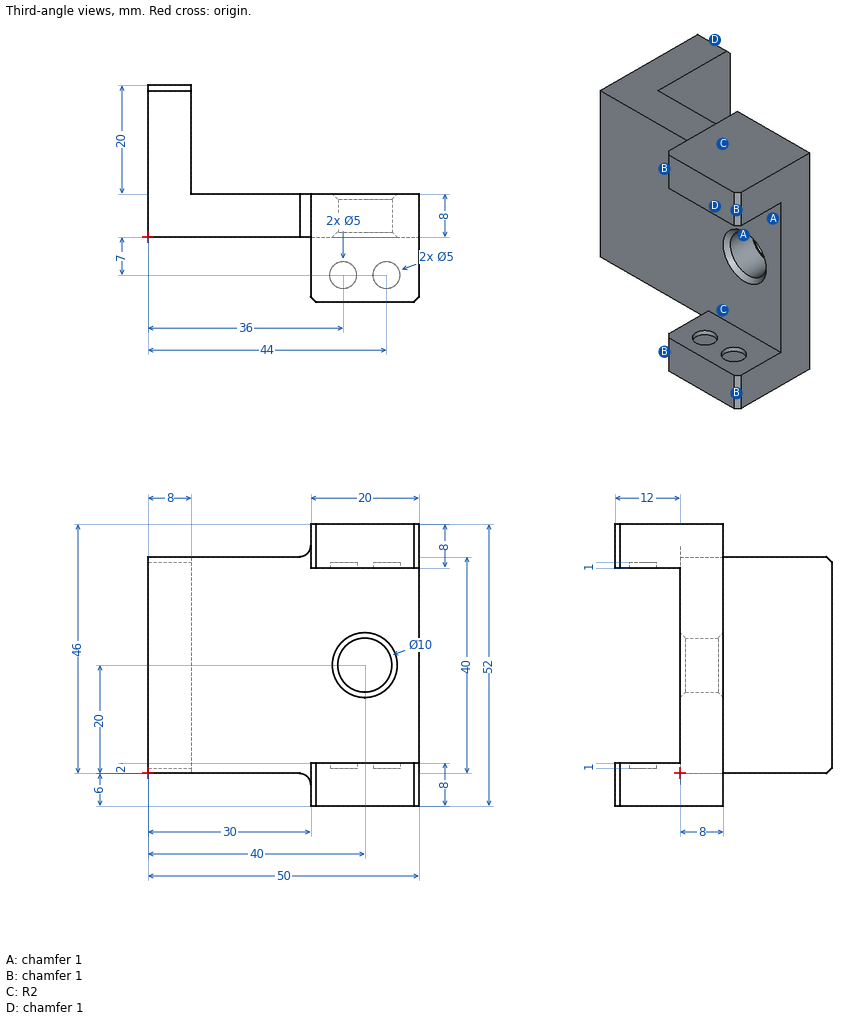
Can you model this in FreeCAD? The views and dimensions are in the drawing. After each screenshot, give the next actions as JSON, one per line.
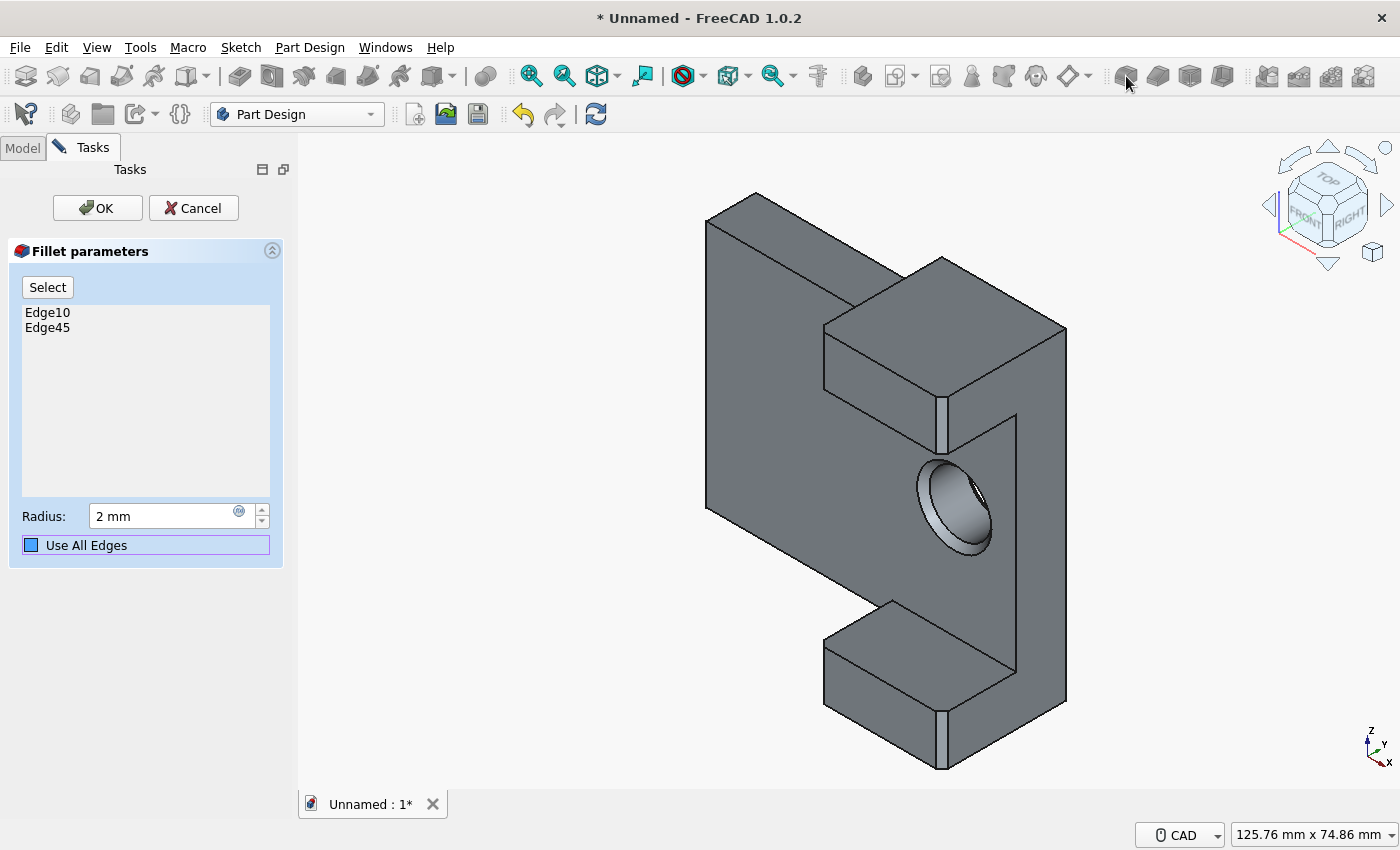
{"action": "left_click", "coordinate": [98, 208]}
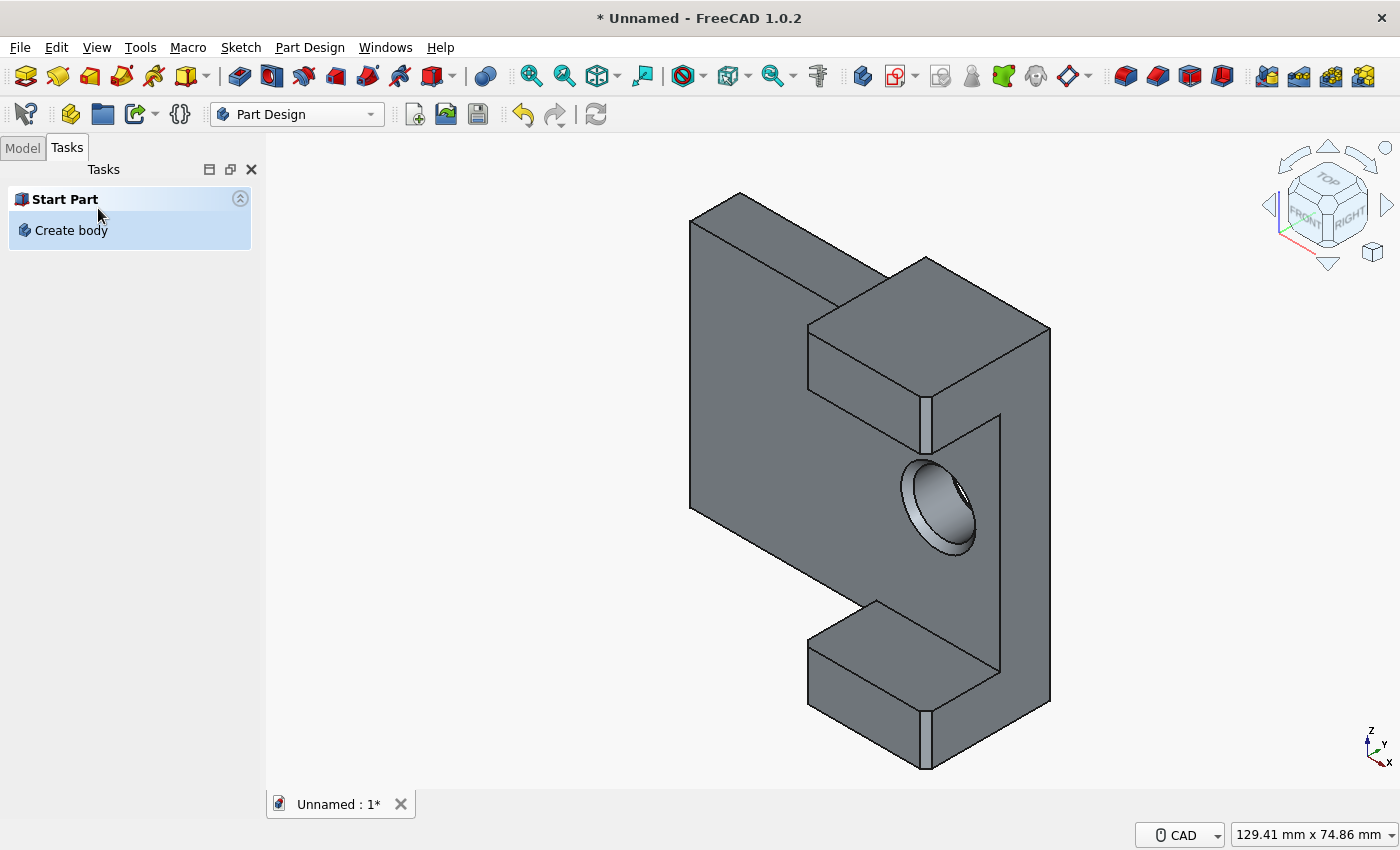
{"action": "key", "text": "4"}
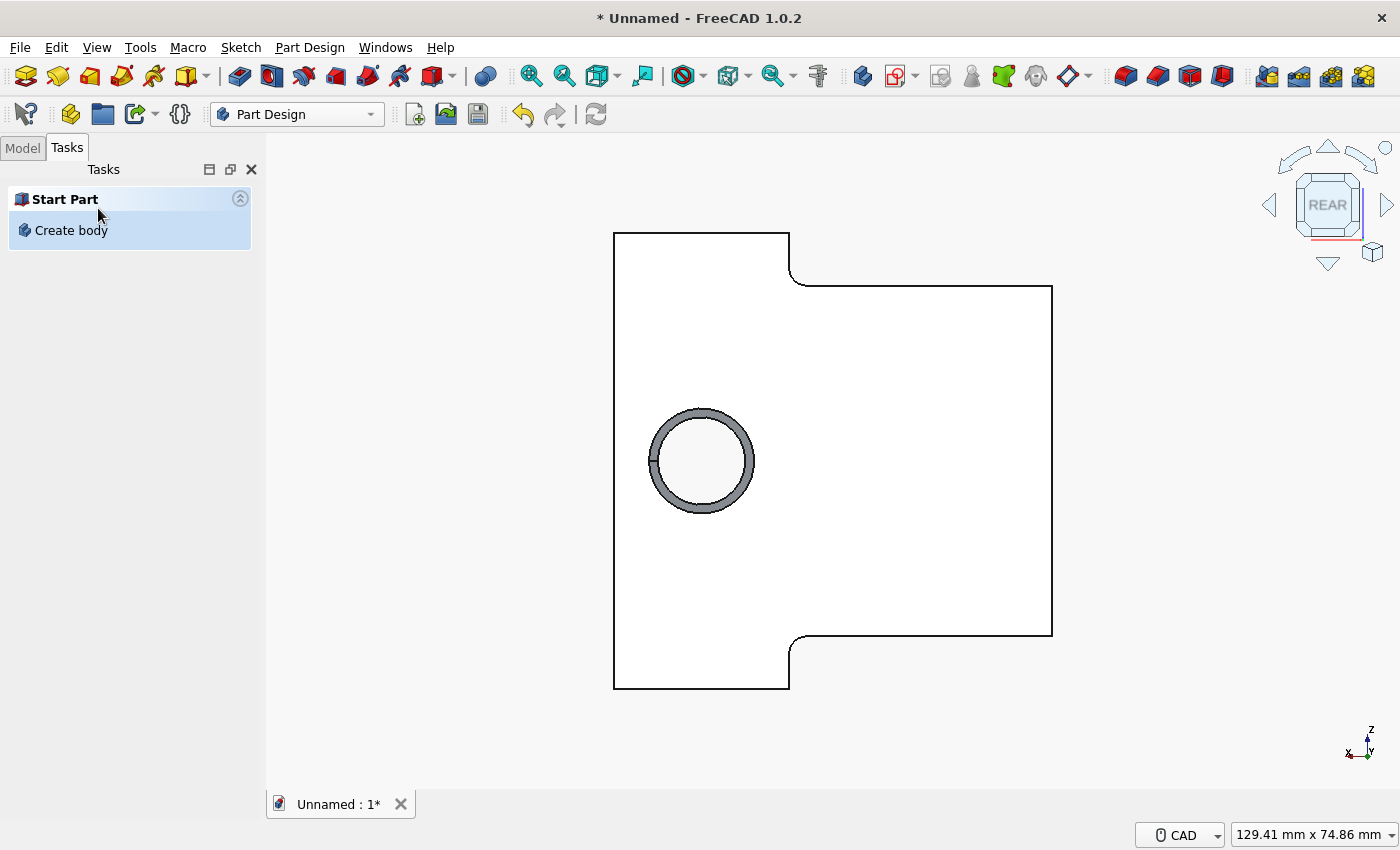
{"action": "left_click", "coordinate": [896, 460]}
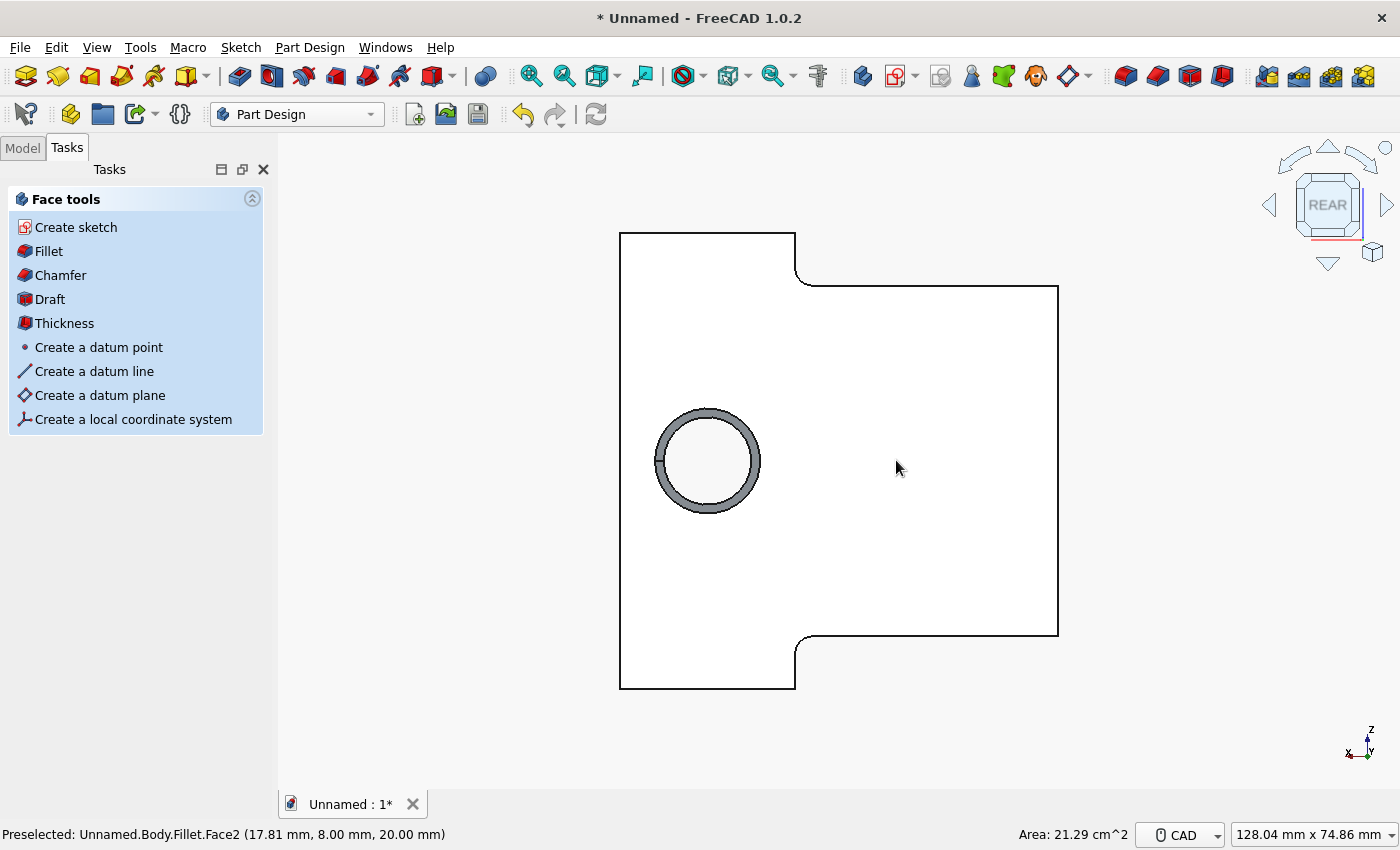
{"action": "left_click", "coordinate": [896, 76]}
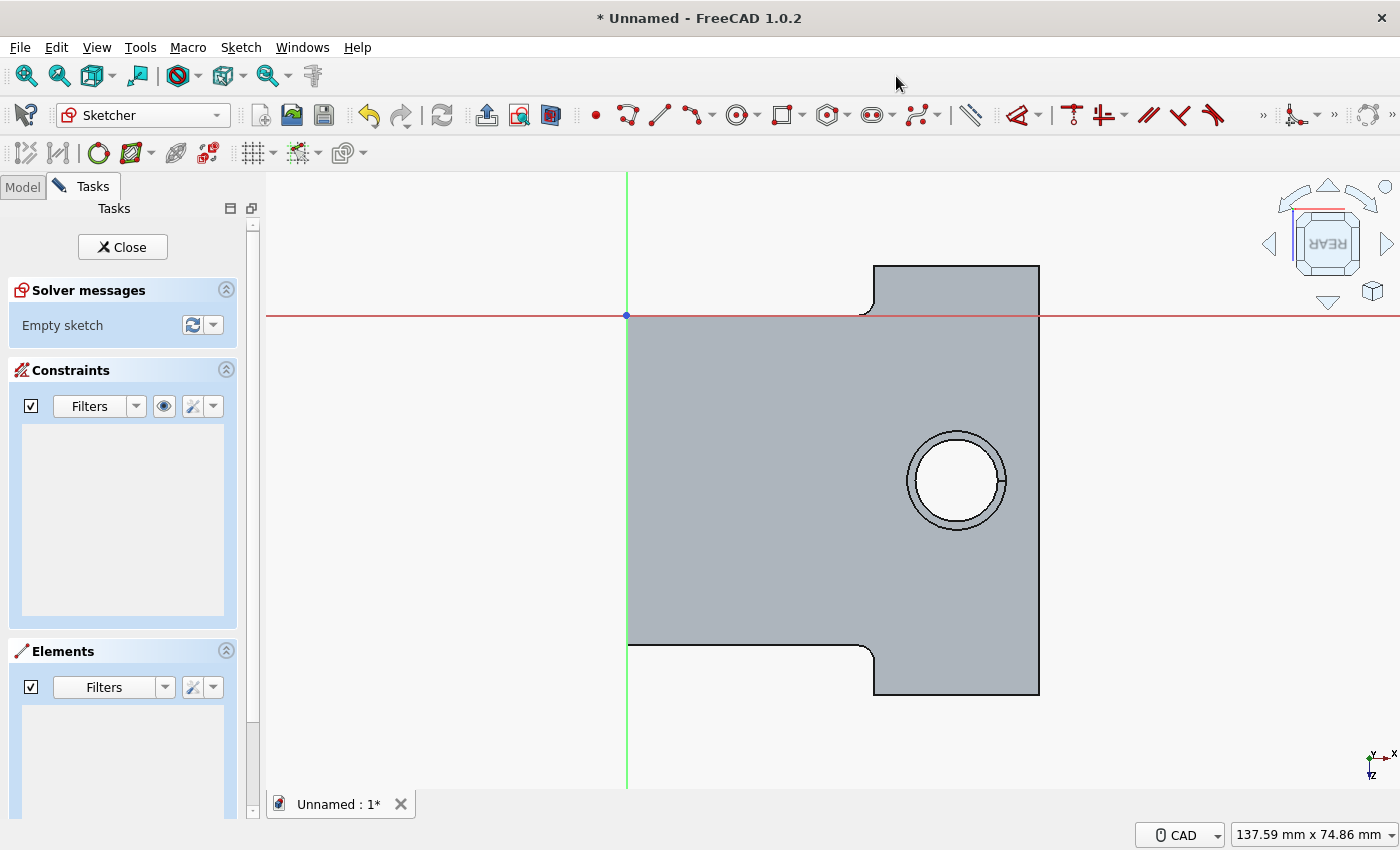
{"action": "key", "text": "g r"}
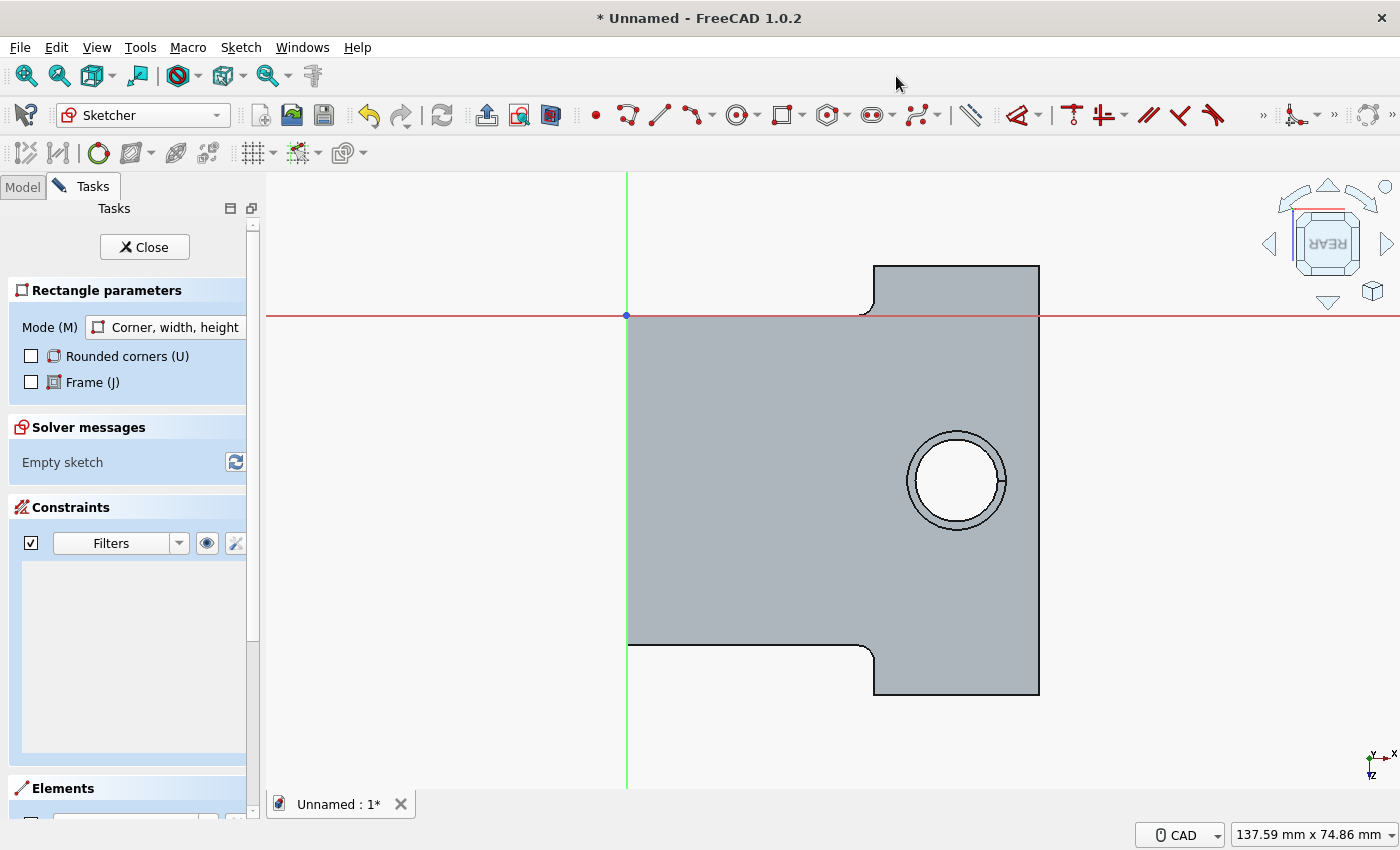
{"action": "left_click", "coordinate": [627, 316]}
{"action": "mouse_move", "coordinate": [693, 645]}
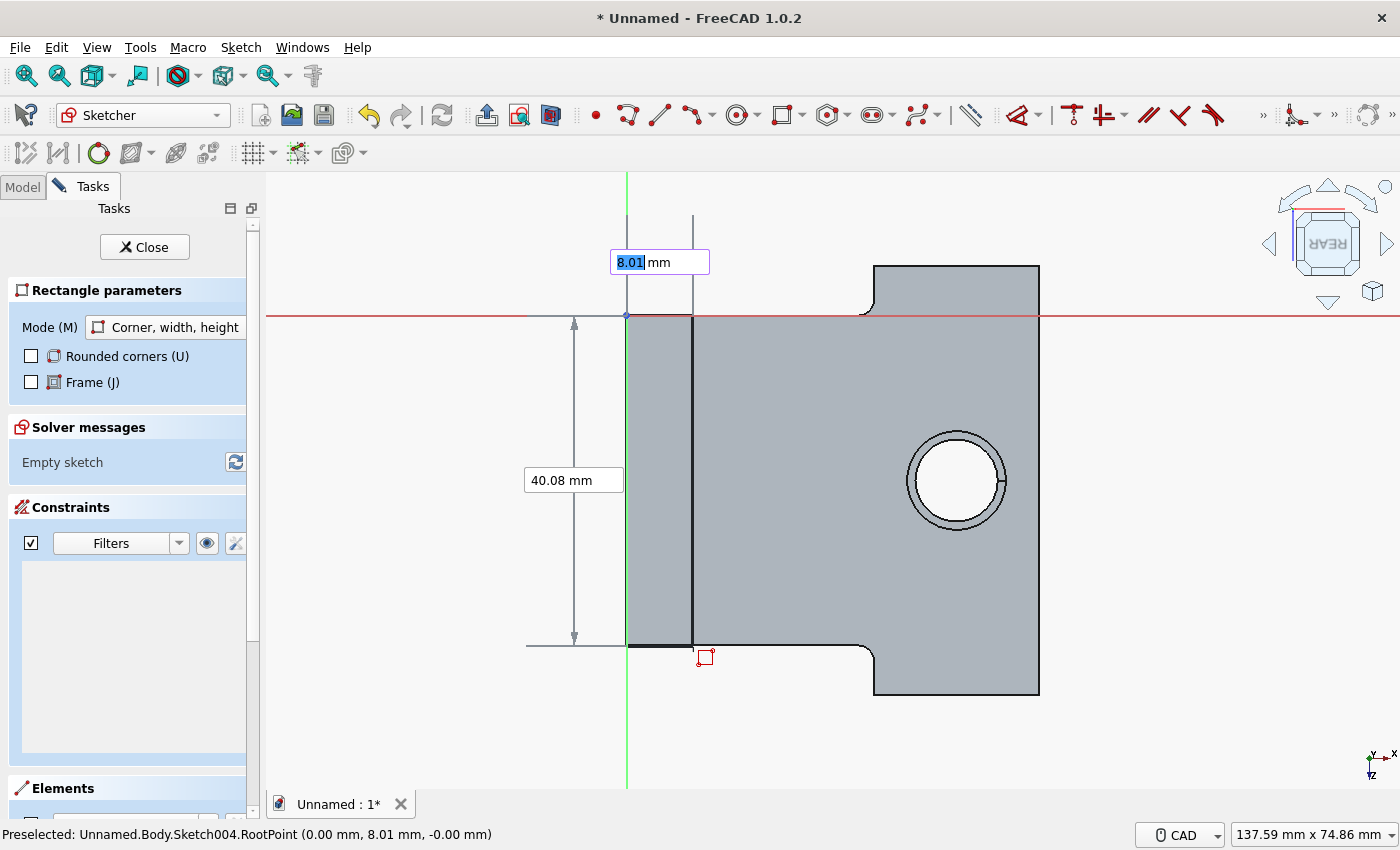
{"action": "type", "text": "8"}
{"action": "key", "text": "Tab"}
{"action": "type", "text": "40"}
{"action": "key", "text": "Return"}
{"action": "key", "text": "Escape"}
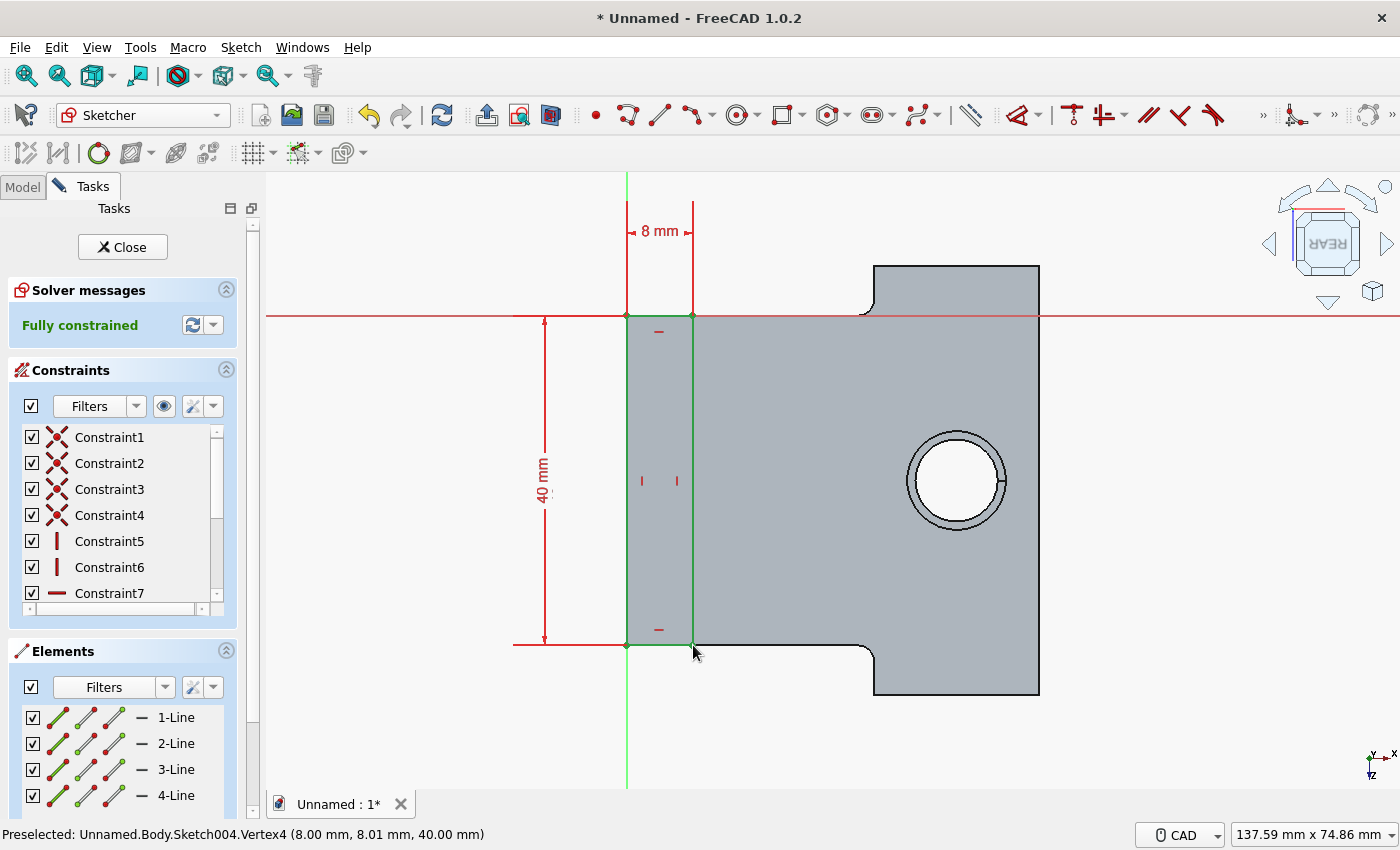
{"action": "left_click", "coordinate": [123, 247]}